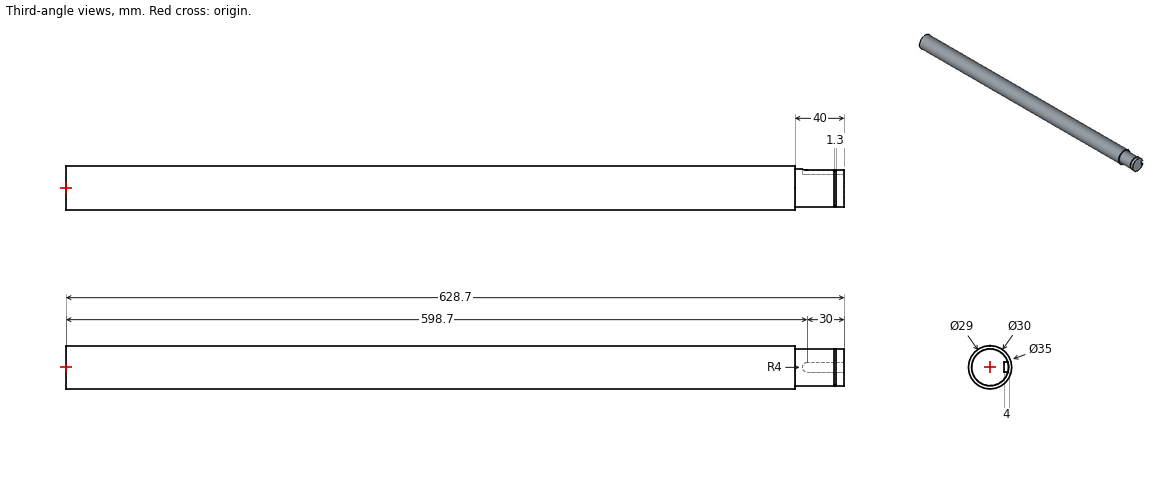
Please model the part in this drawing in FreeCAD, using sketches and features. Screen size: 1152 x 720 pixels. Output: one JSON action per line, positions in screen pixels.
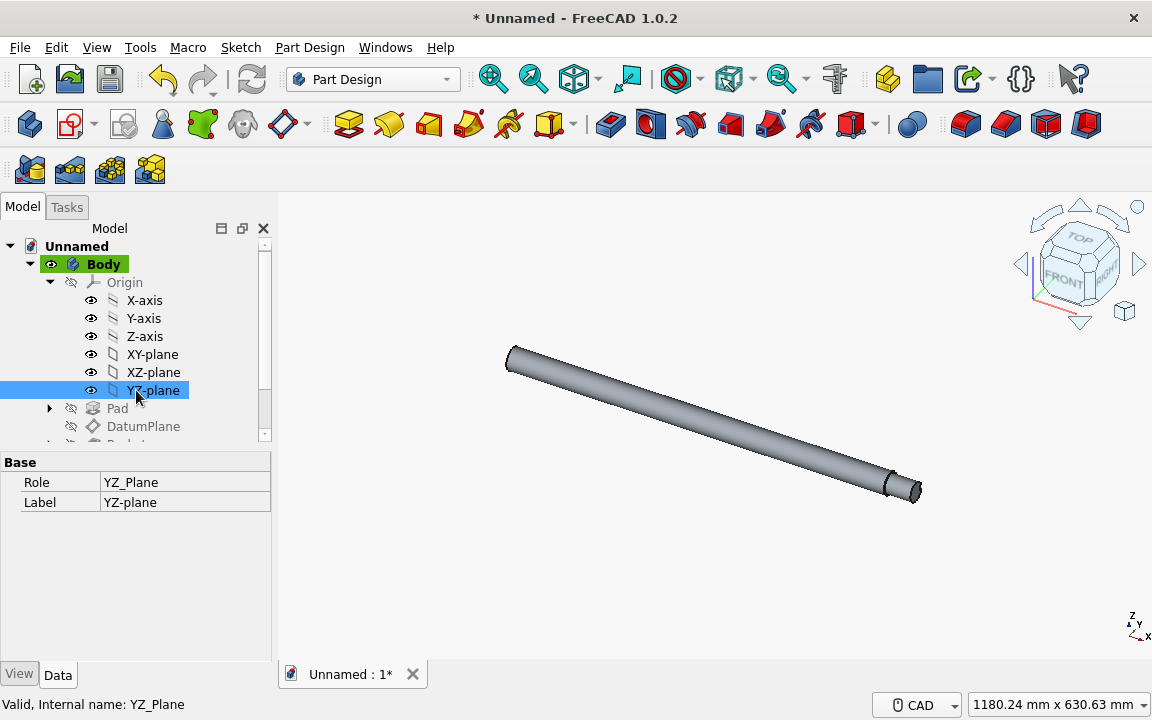
{"action": "left_click", "coordinate": [284, 124]}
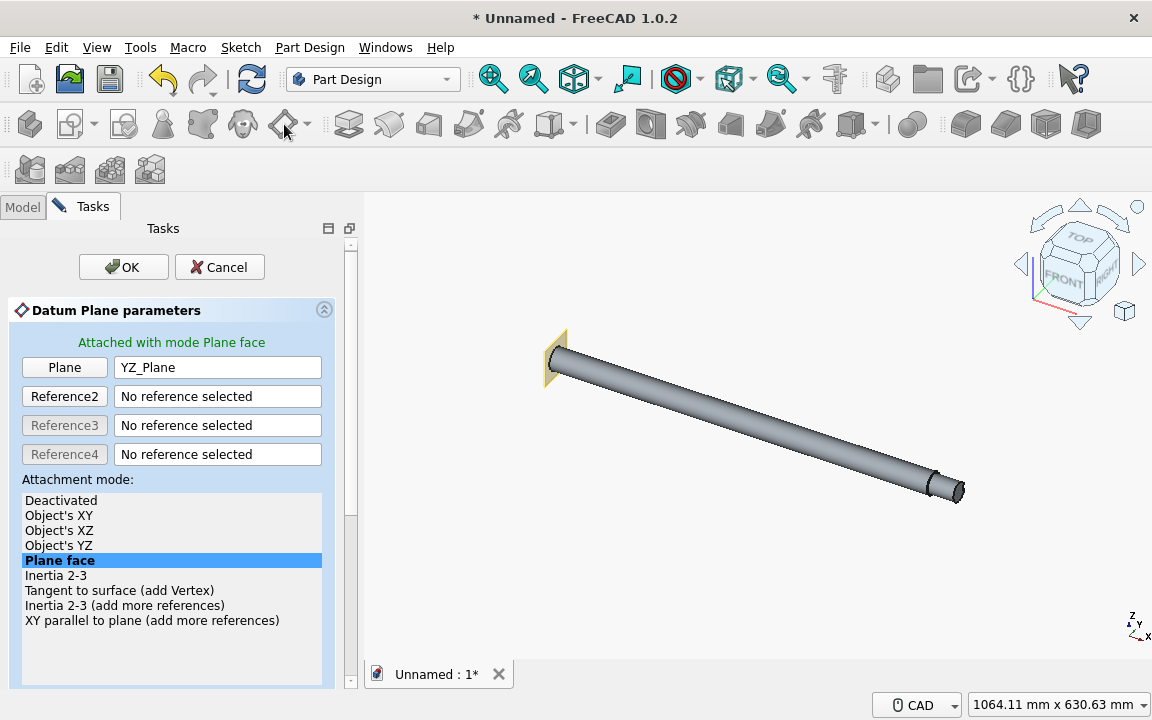
{"action": "scroll", "coordinate": [351, 463], "scroll_direction": "down", "scroll_amount": 3}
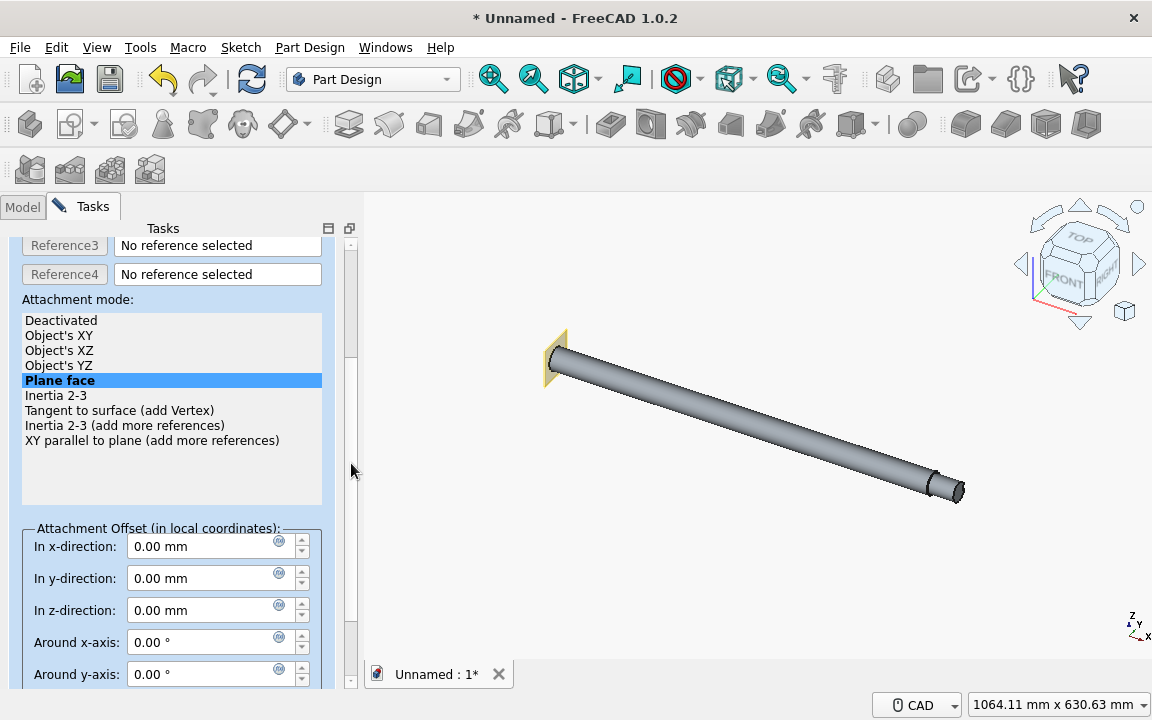
{"action": "triple_click", "coordinate": [210, 610]}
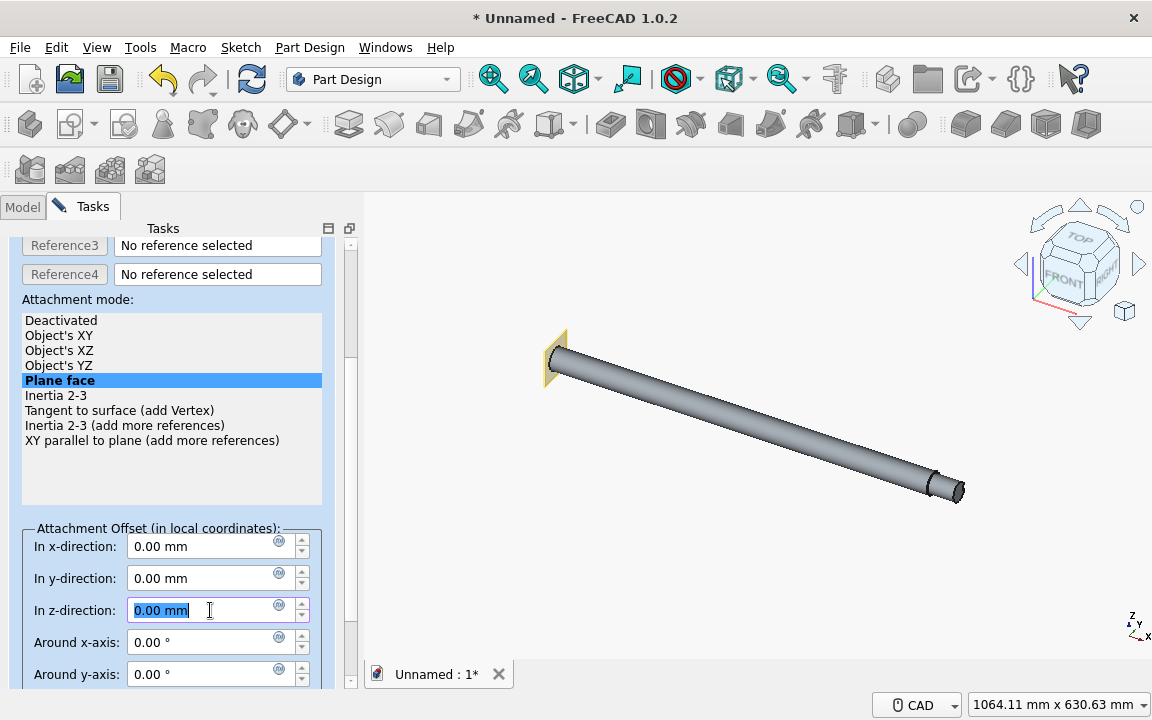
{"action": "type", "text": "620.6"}
{"action": "key", "text": "Tab"}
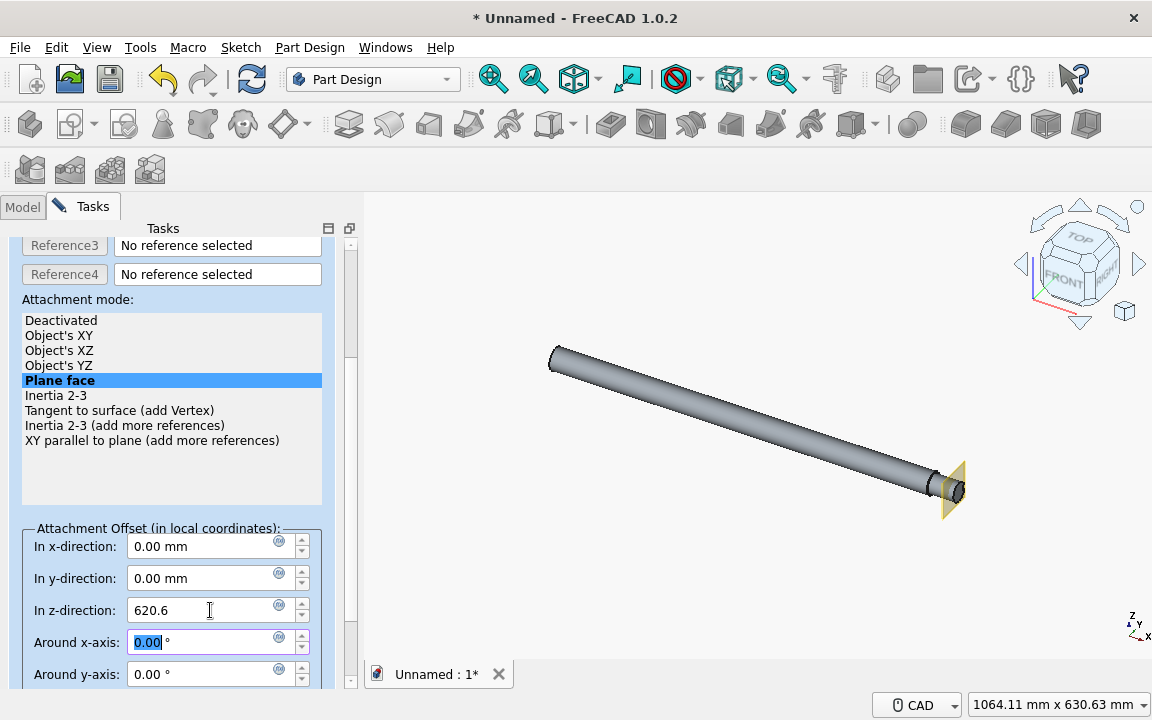
{"action": "scroll", "coordinate": [351, 463], "scroll_direction": "up", "scroll_amount": 4}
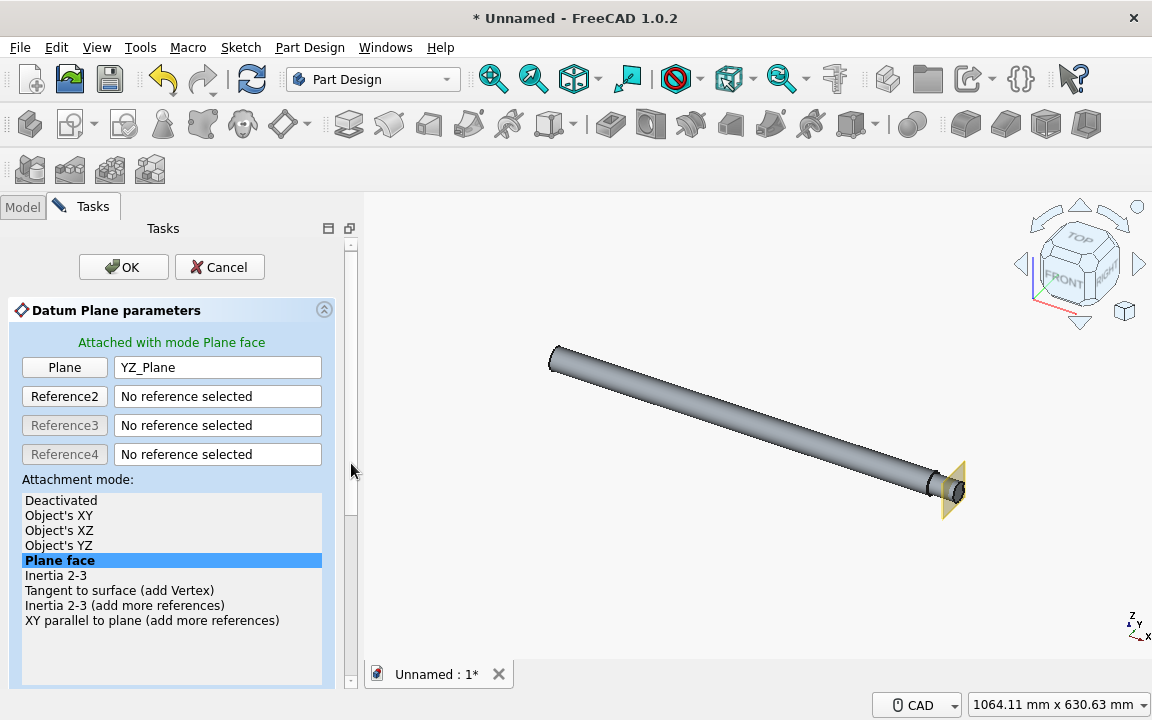
{"action": "left_click", "coordinate": [124, 267]}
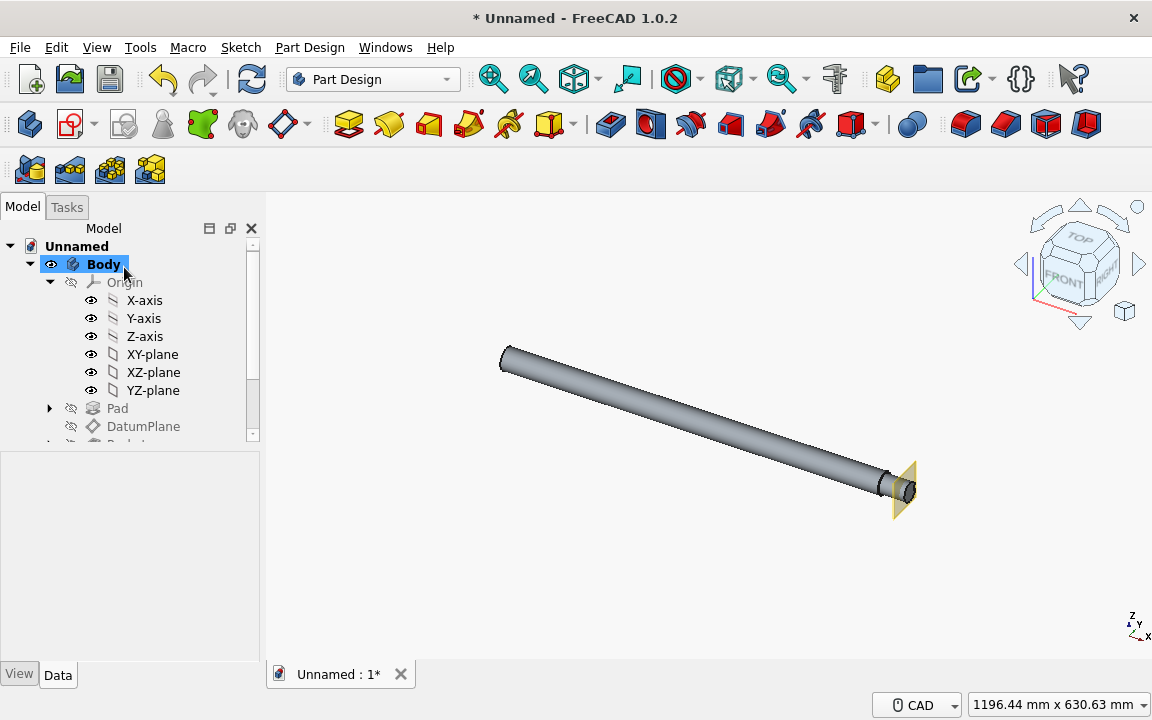
{"action": "scroll", "coordinate": [100, 332], "scroll_direction": "down", "scroll_amount": 3}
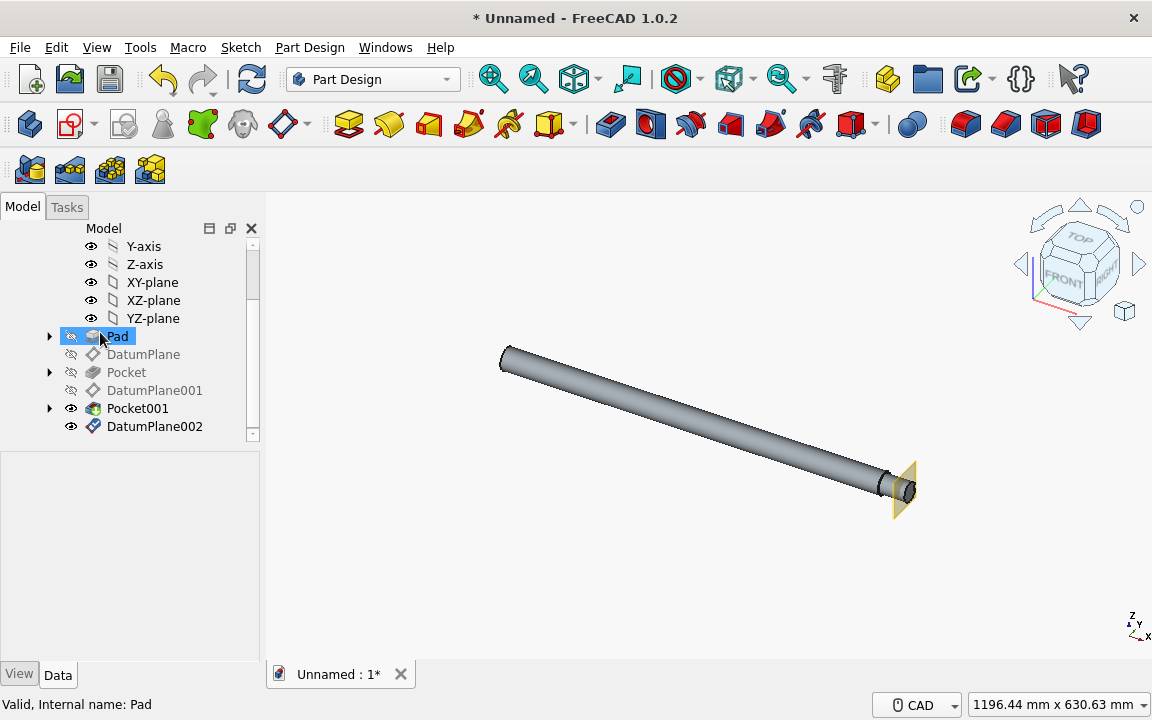
{"action": "left_click", "coordinate": [116, 426]}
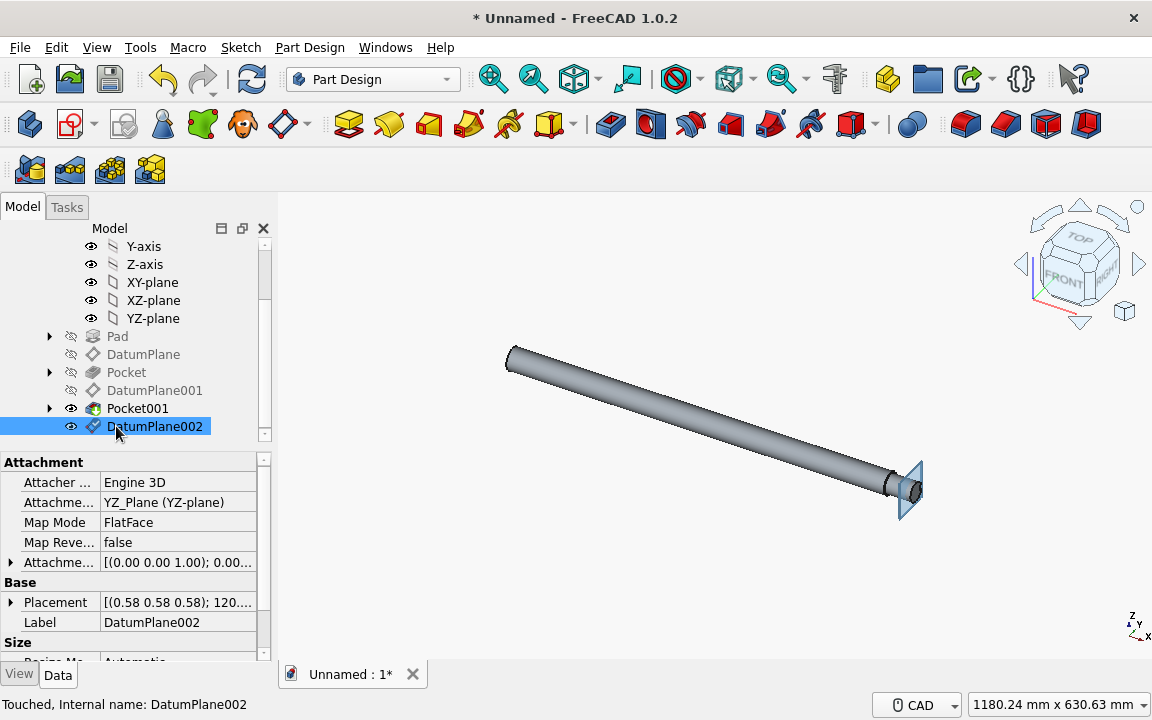
{"action": "left_click", "coordinate": [70, 124]}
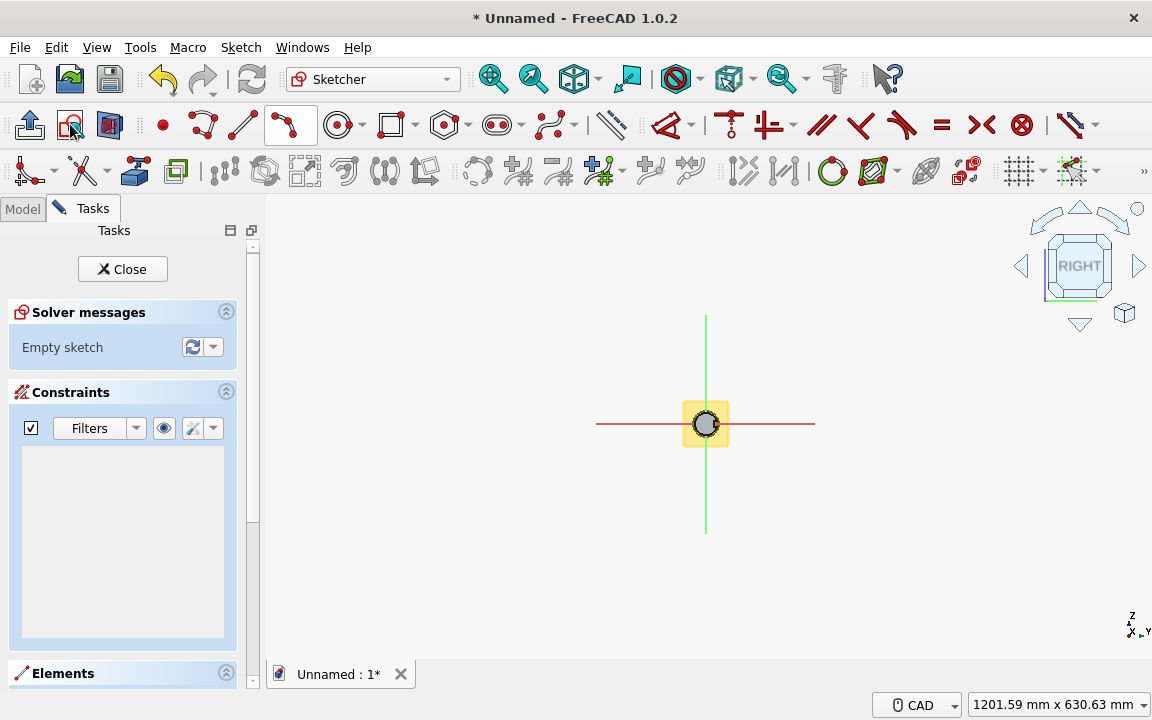
{"action": "key", "text": "q s"}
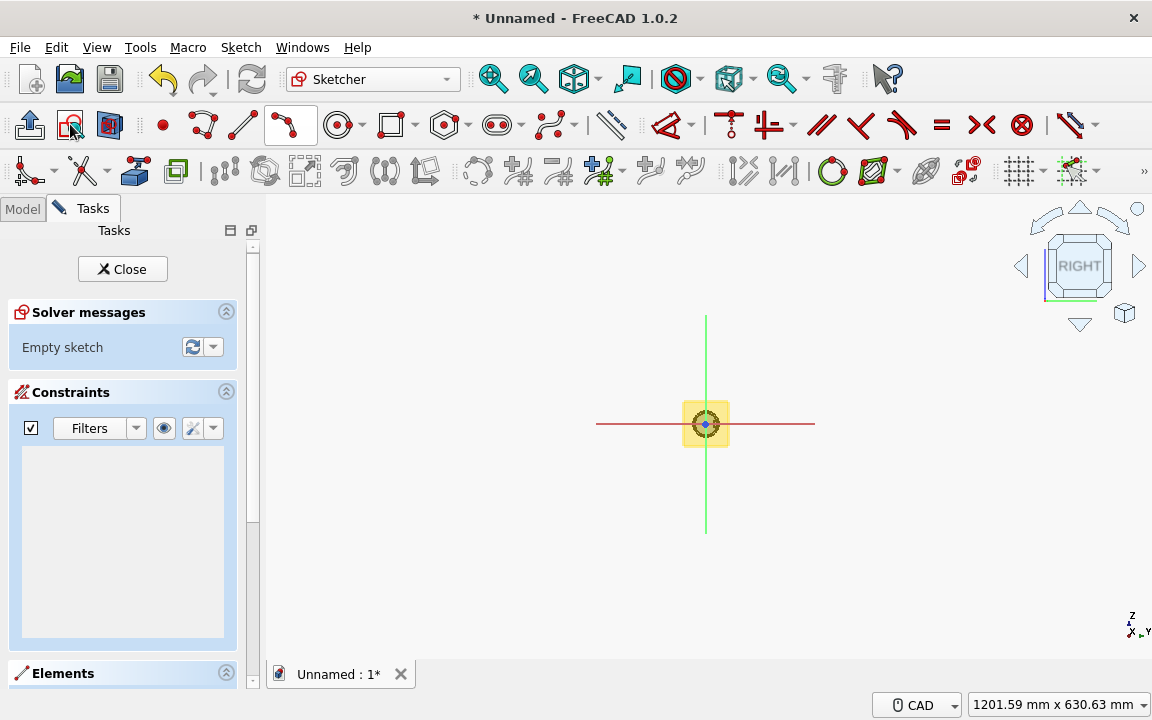
{"action": "scroll", "coordinate": [711, 424], "scroll_direction": "up", "scroll_amount": 13}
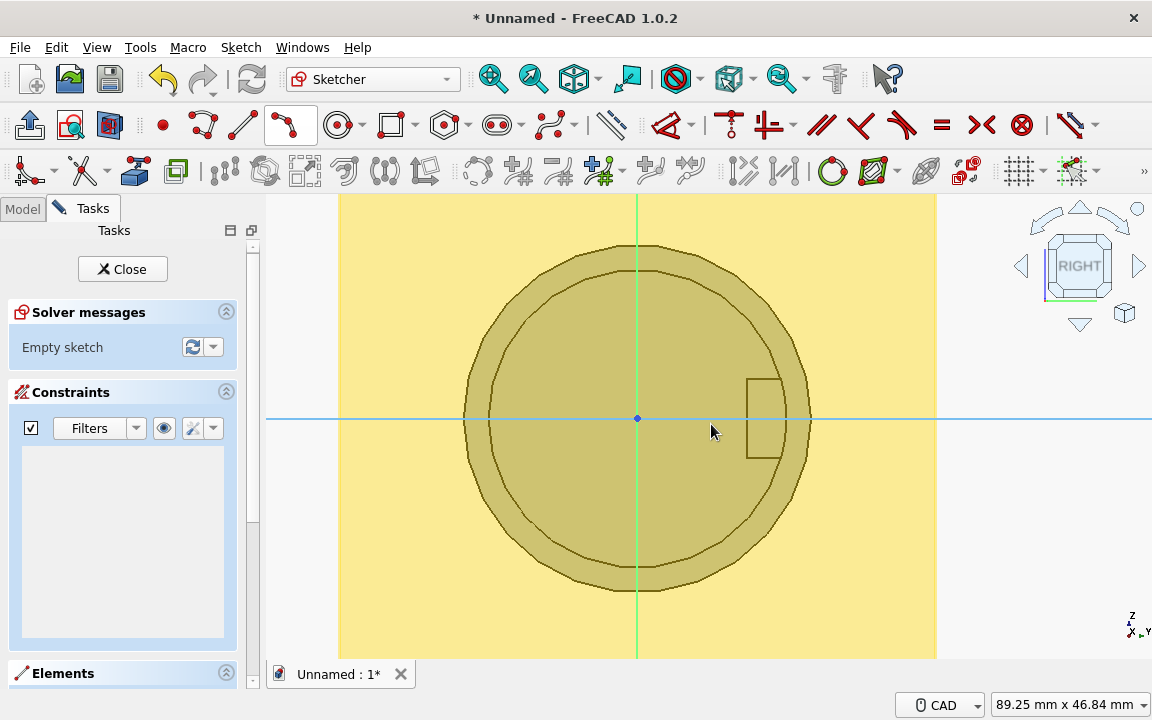
{"action": "left_click", "coordinate": [338, 126]}